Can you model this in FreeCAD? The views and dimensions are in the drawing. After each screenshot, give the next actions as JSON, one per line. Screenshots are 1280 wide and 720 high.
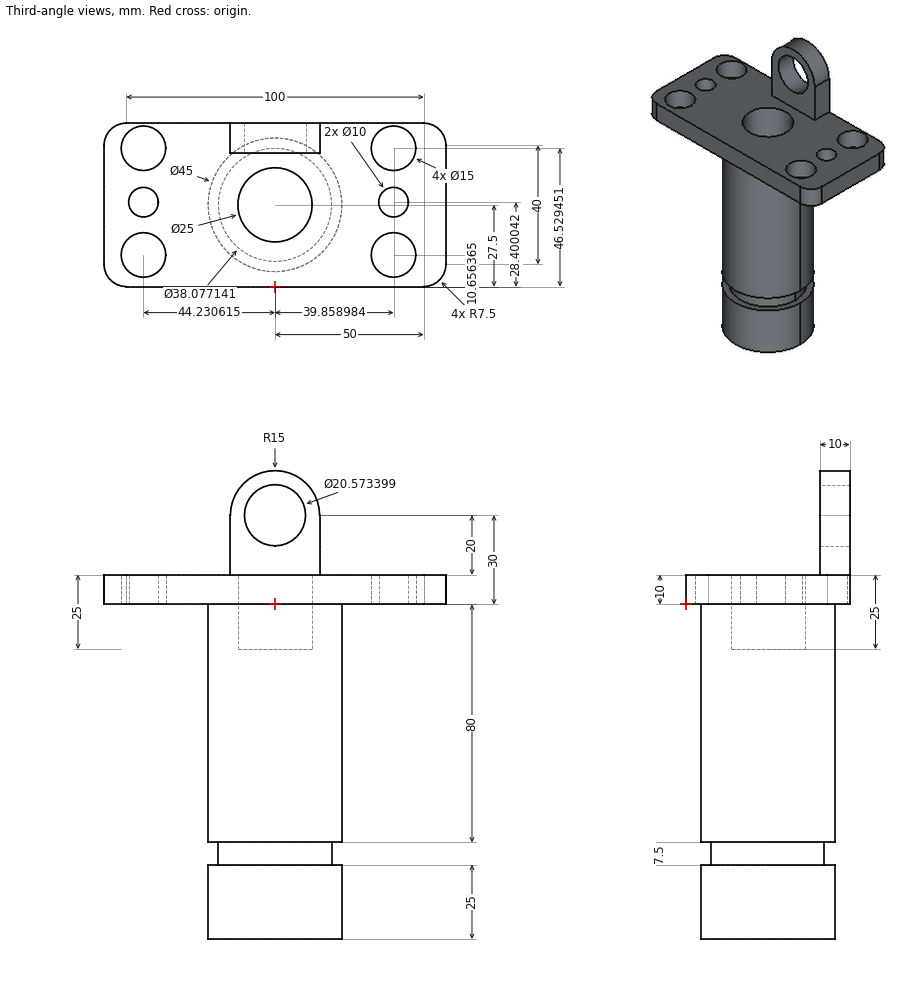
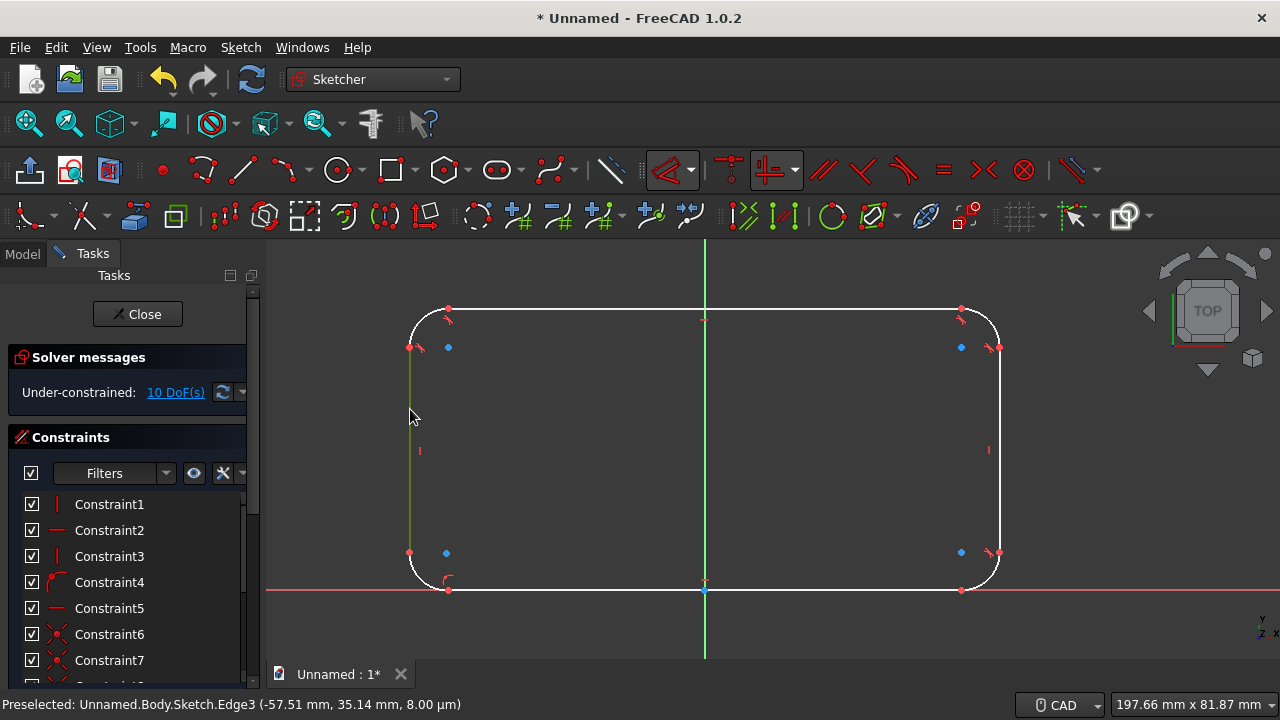
{"action": "left_click", "coordinate": [414, 570]}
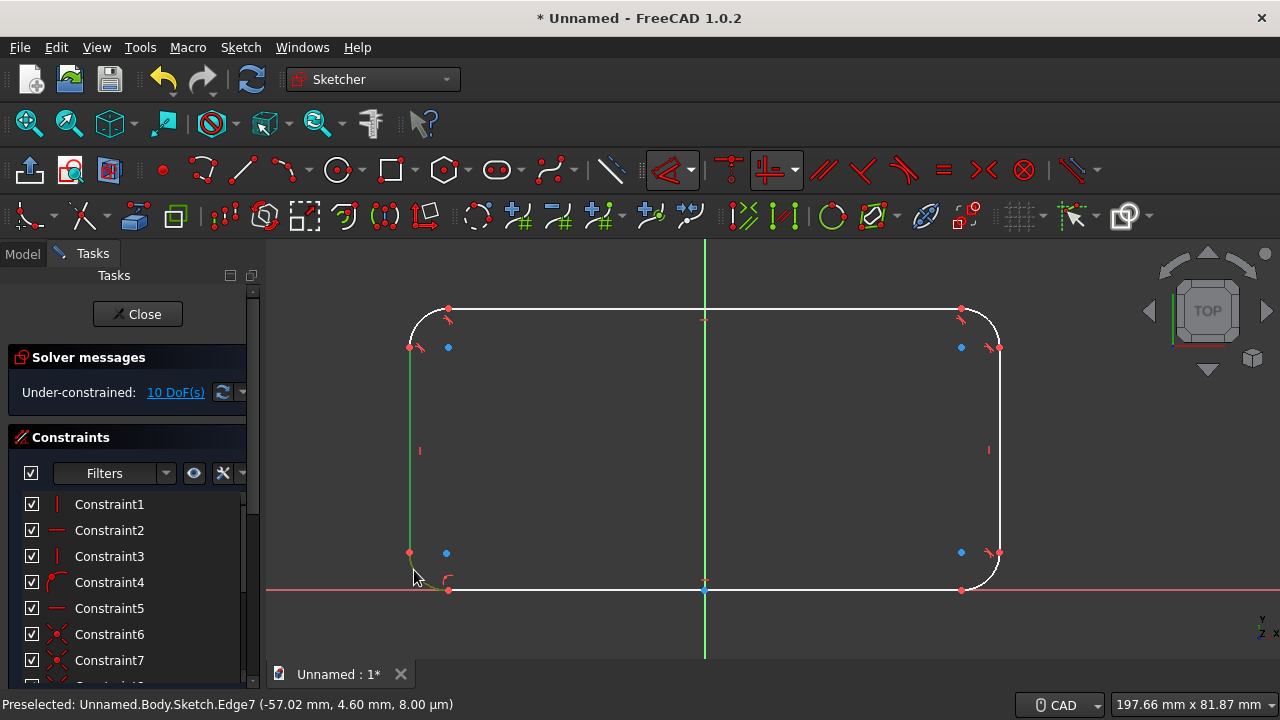
{"action": "left_click", "coordinate": [904, 170]}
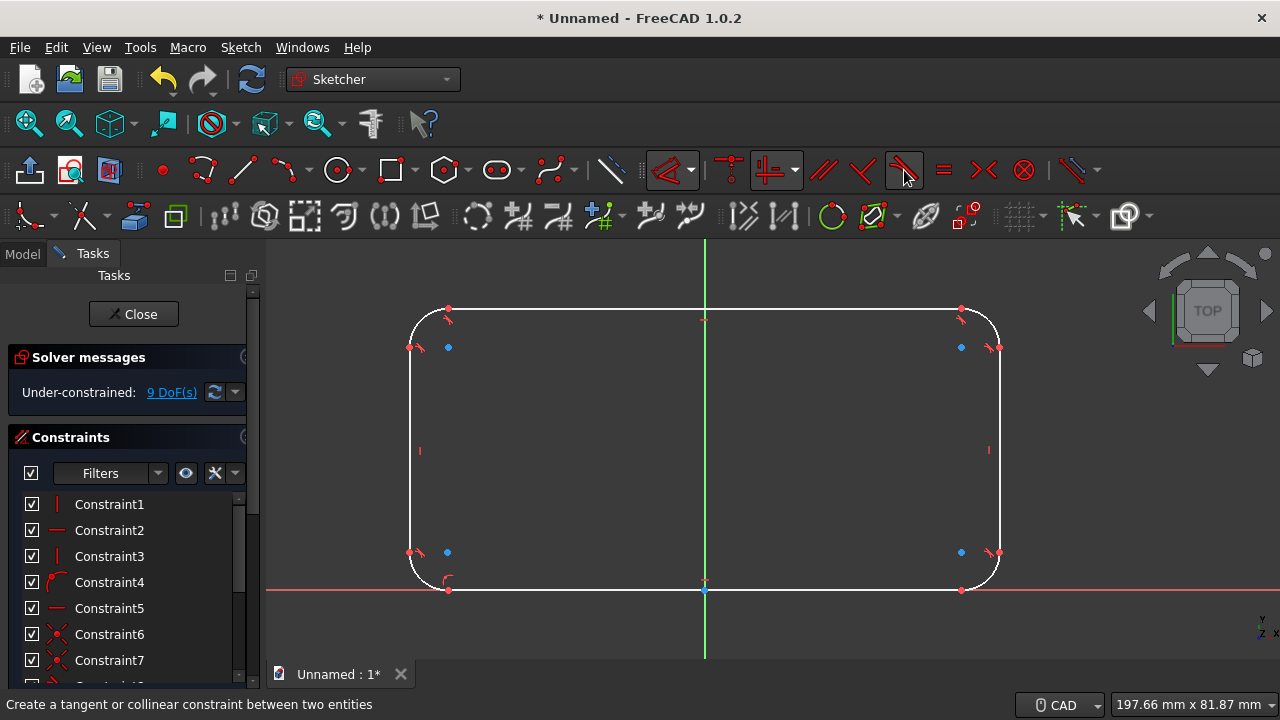
{"action": "left_click", "coordinate": [603, 590]}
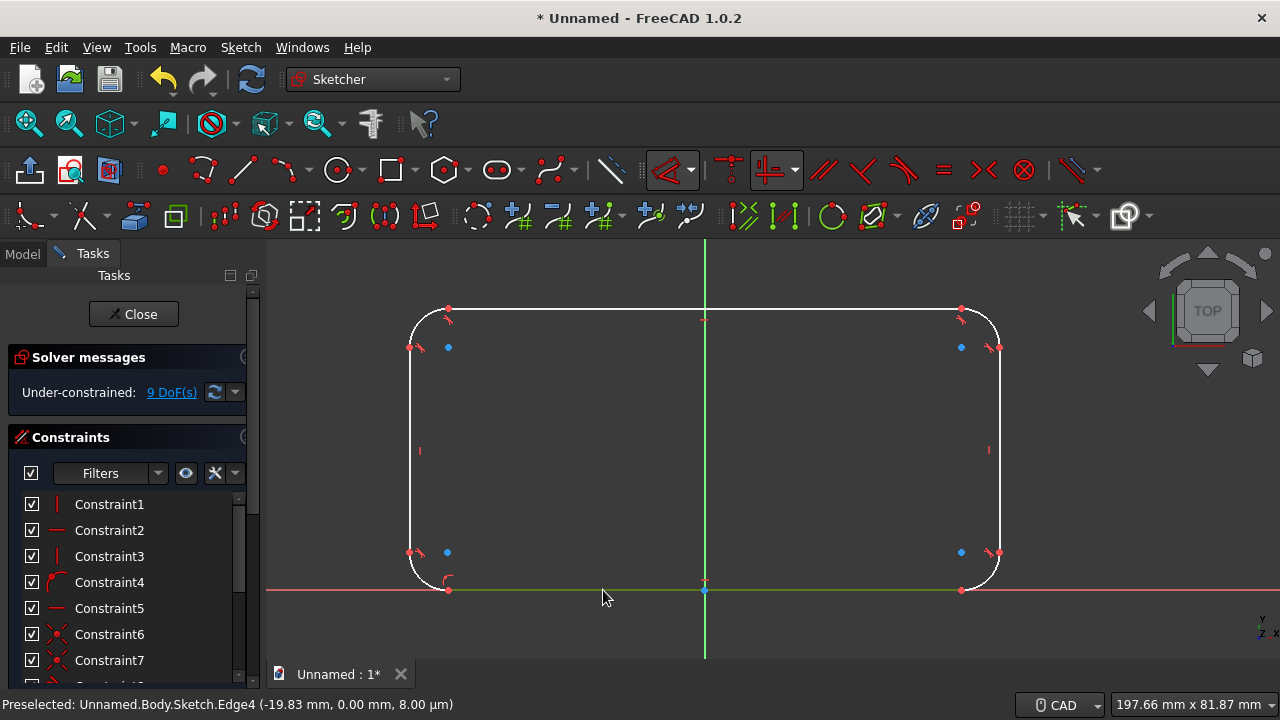
{"action": "left_click", "coordinate": [414, 570]}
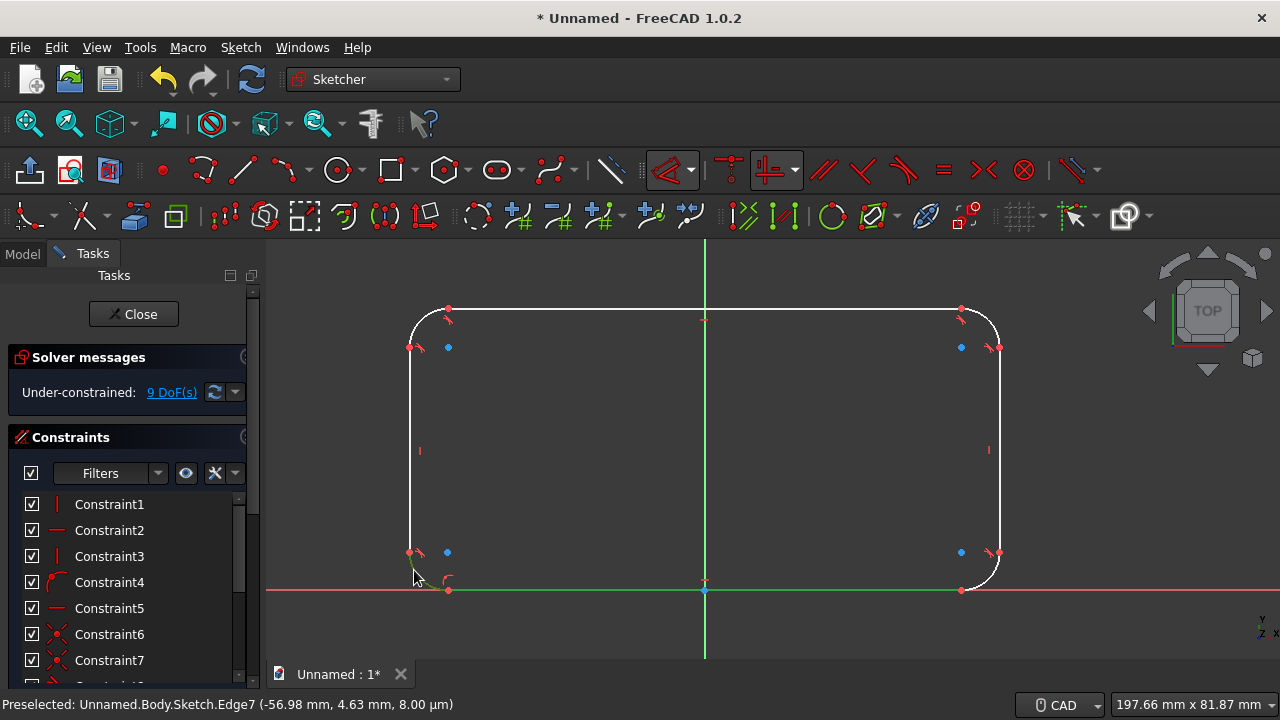
{"action": "left_click", "coordinate": [904, 170]}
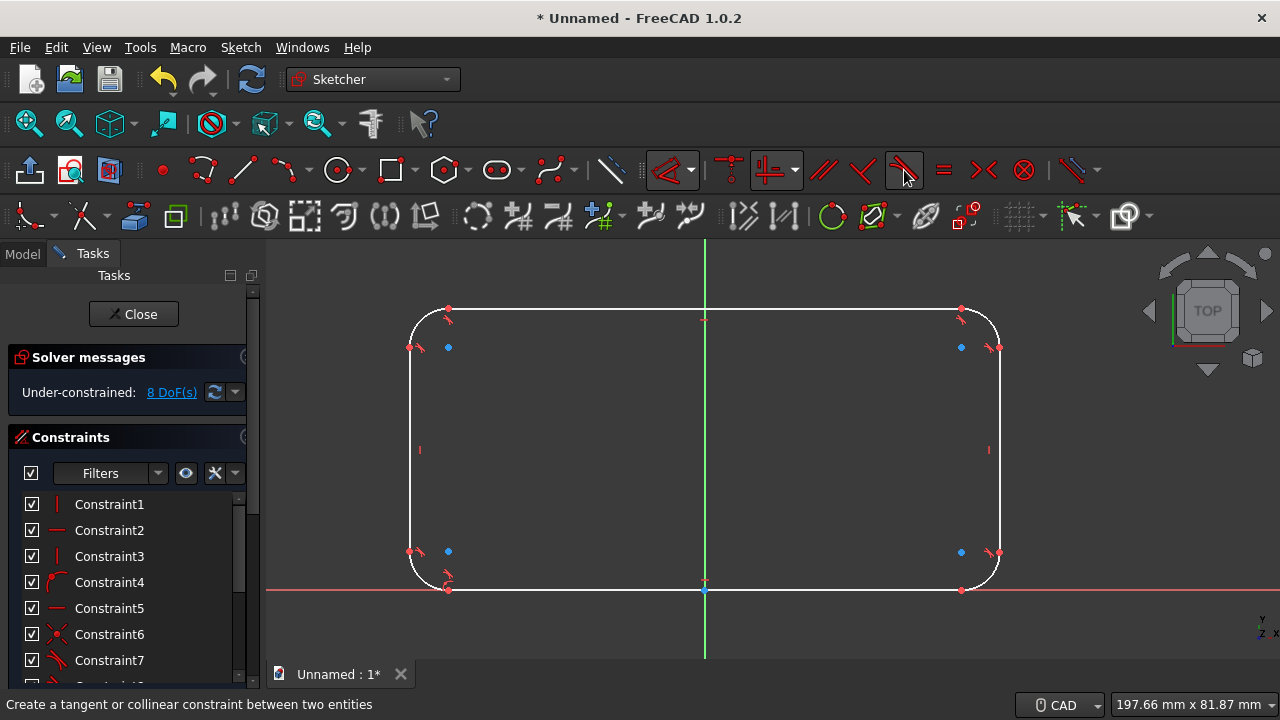
{"action": "left_click", "coordinate": [603, 590]}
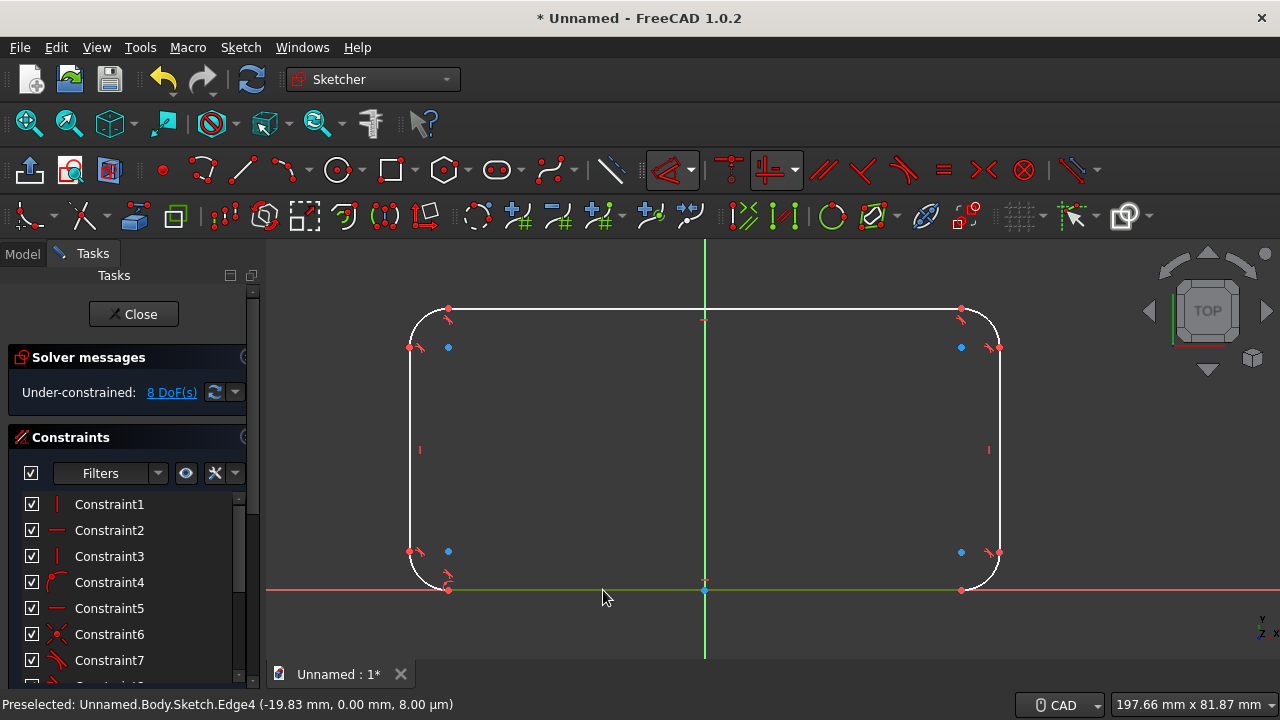
{"action": "left_click", "coordinate": [996, 570]}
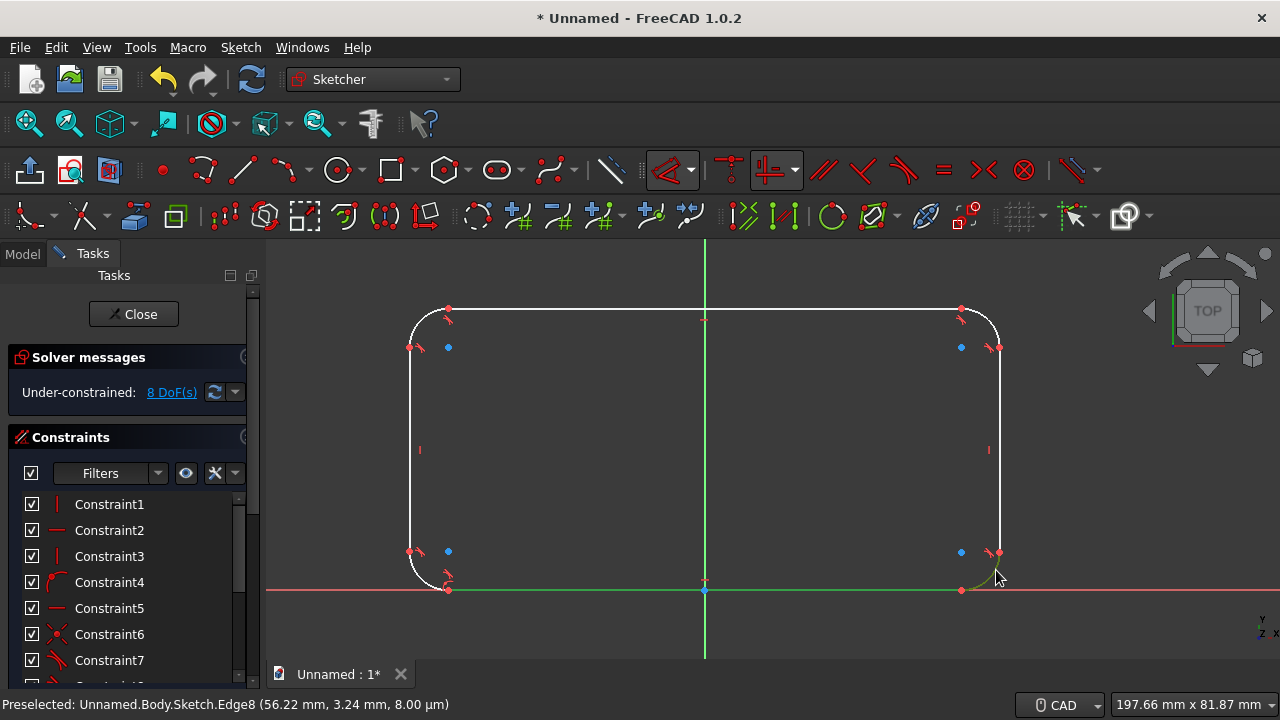
{"action": "left_click", "coordinate": [904, 170]}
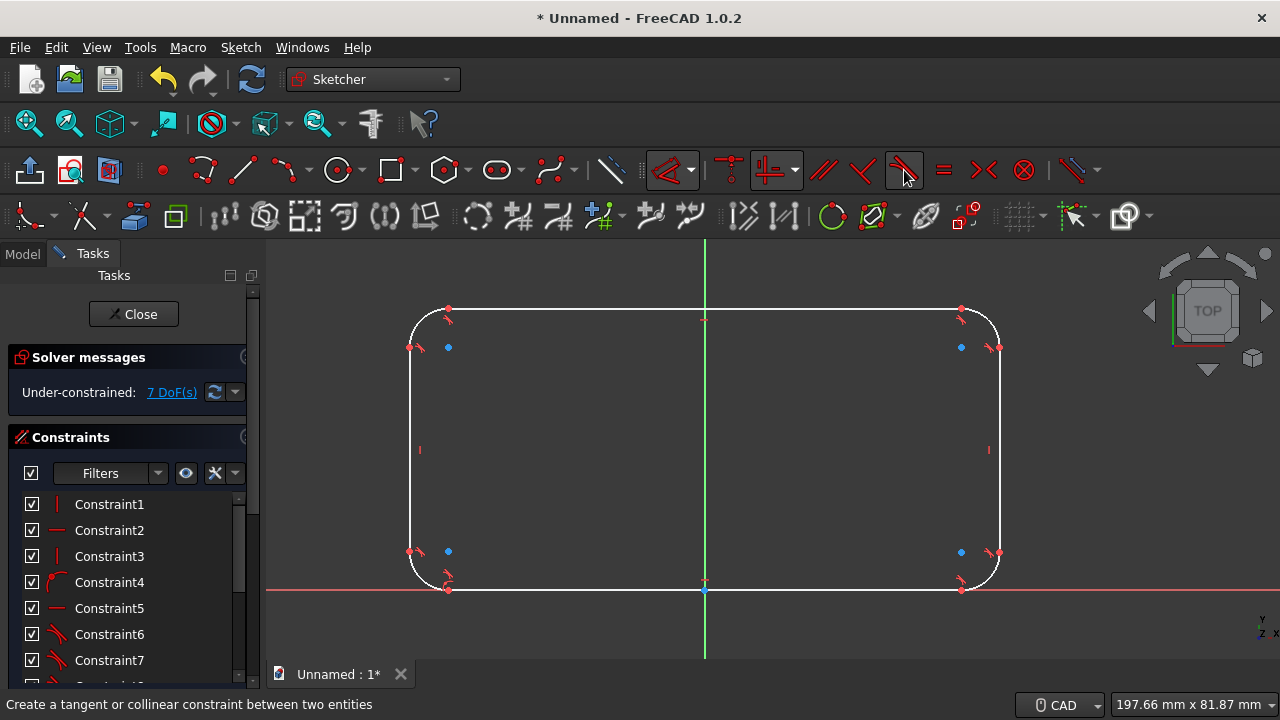
{"action": "left_click", "coordinate": [995, 330]}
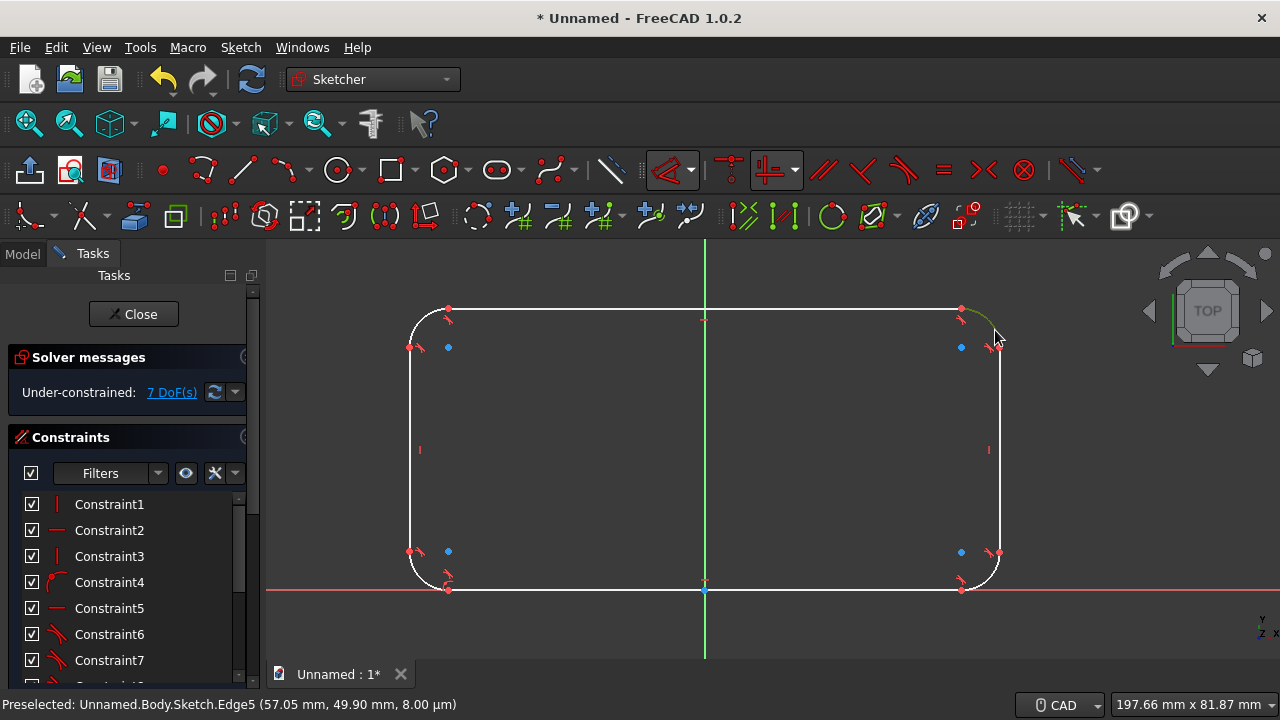
{"action": "left_click", "coordinate": [431, 313]}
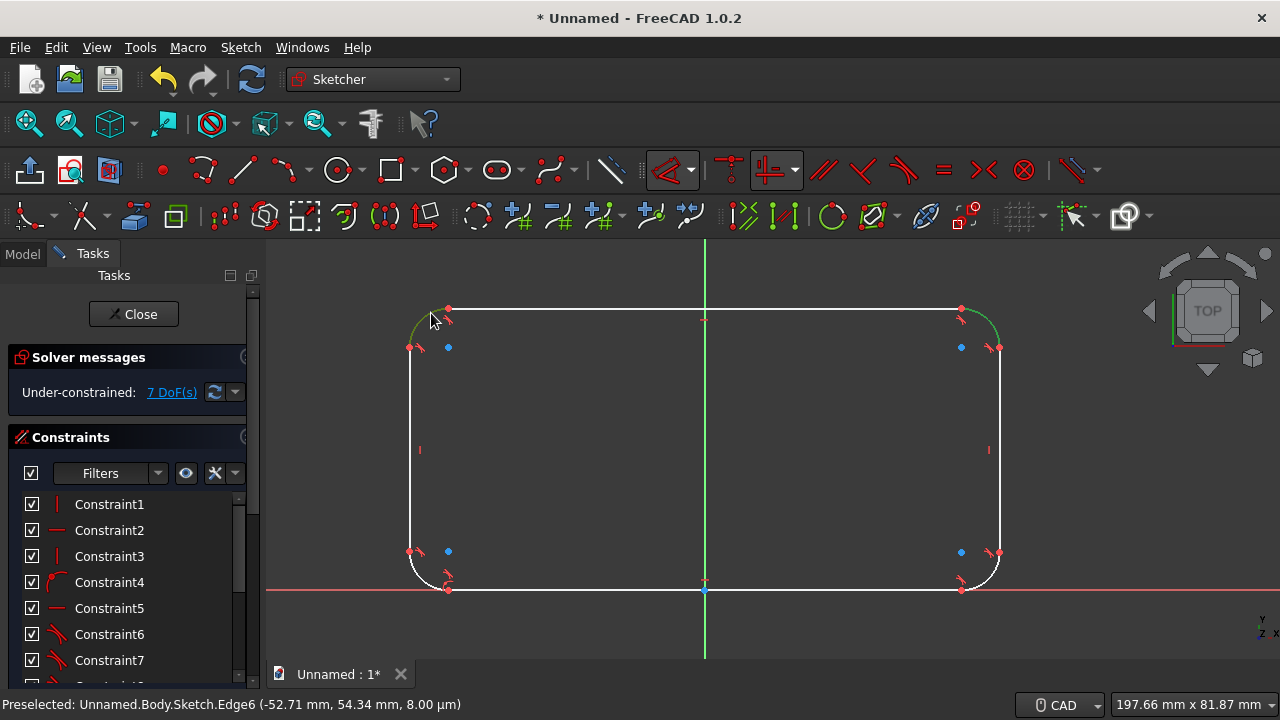
{"action": "left_click", "coordinate": [414, 569]}